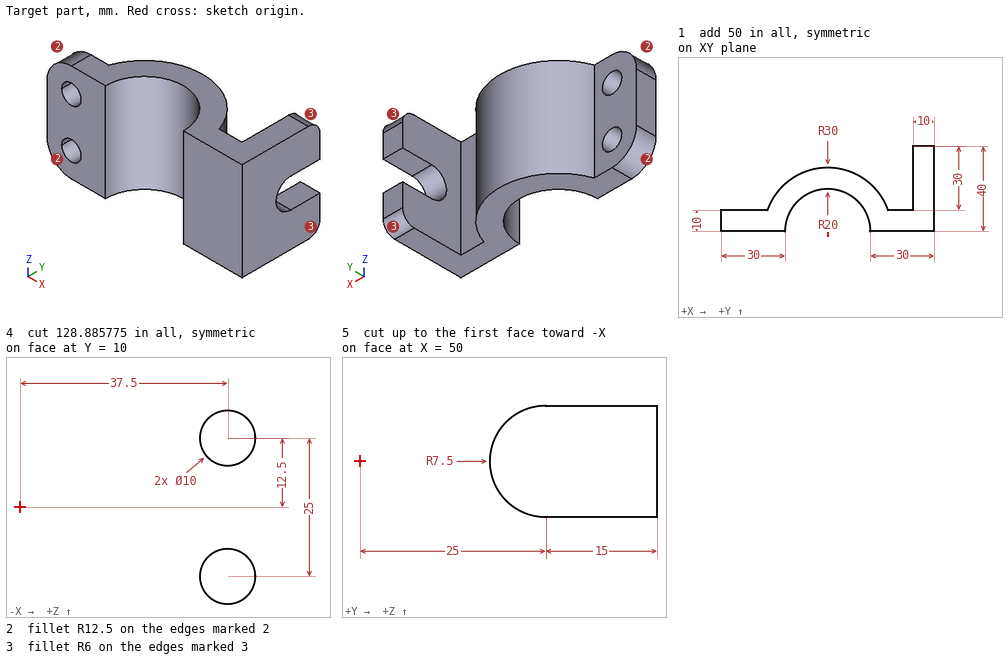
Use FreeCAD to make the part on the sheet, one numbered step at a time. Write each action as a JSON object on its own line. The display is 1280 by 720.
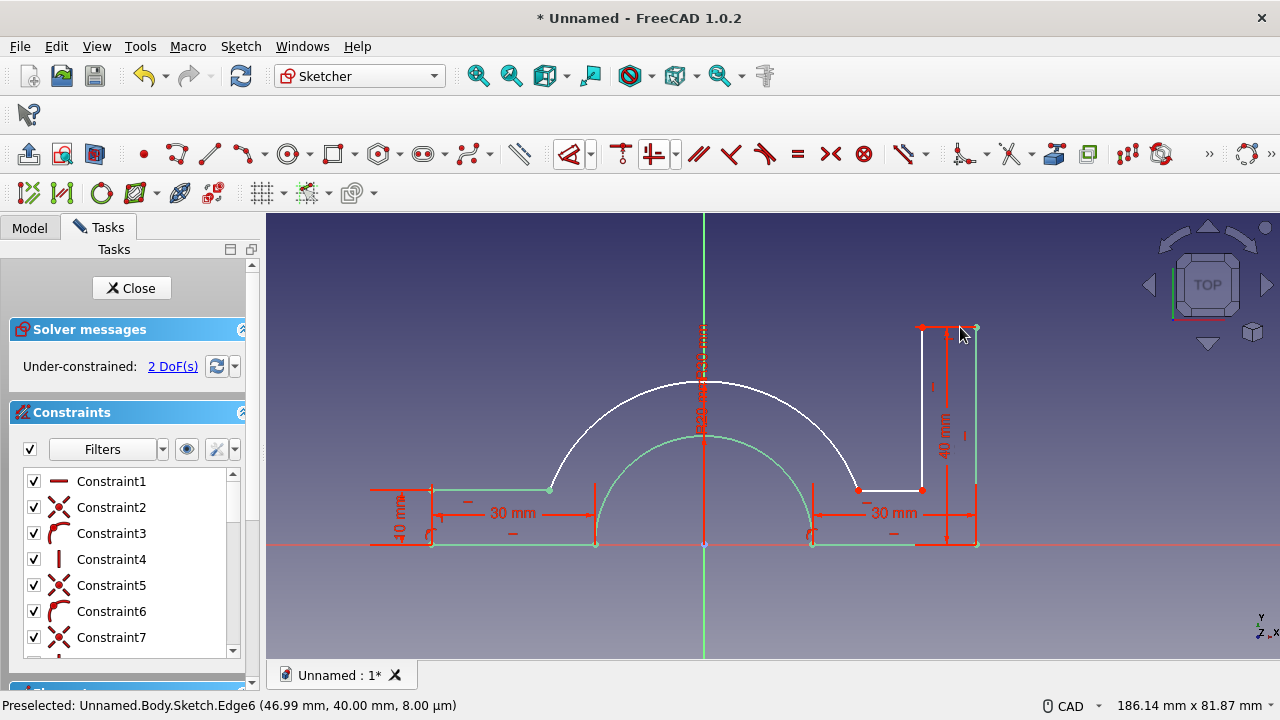
{"action": "key", "text": "l"}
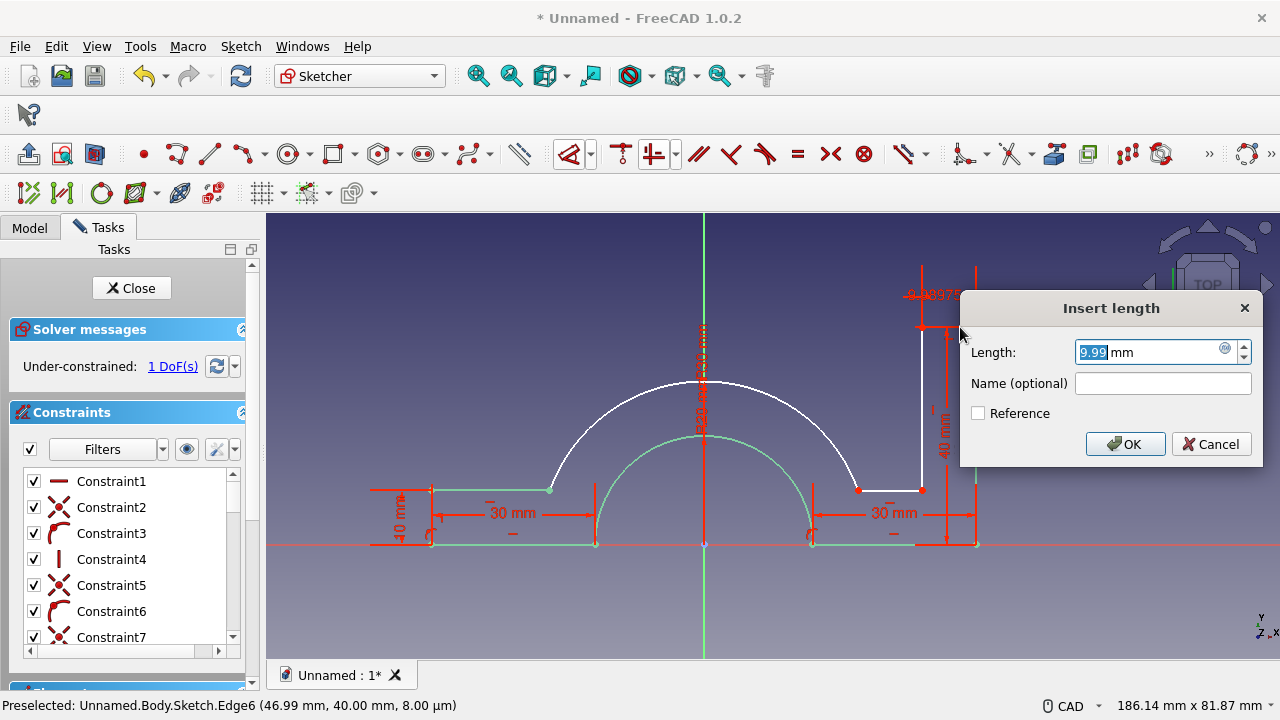
{"action": "type", "text": "10"}
{"action": "key", "text": "Return"}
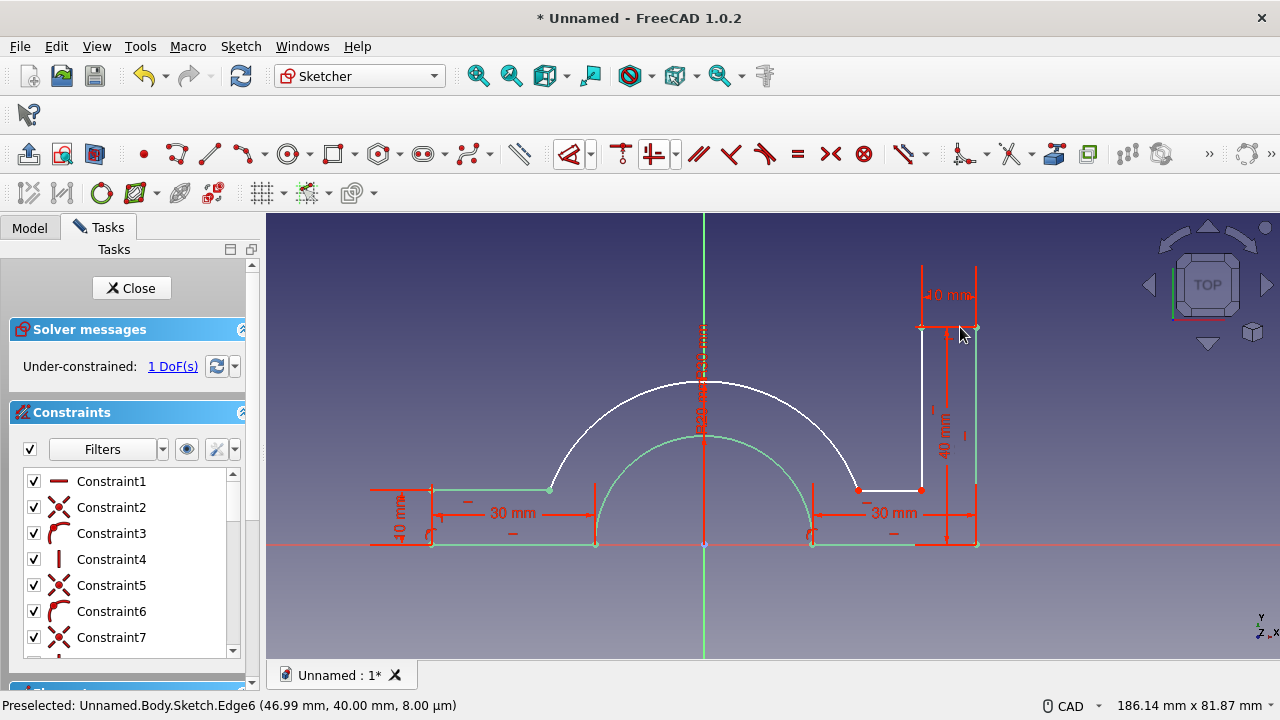
{"action": "left_click", "coordinate": [922, 376]}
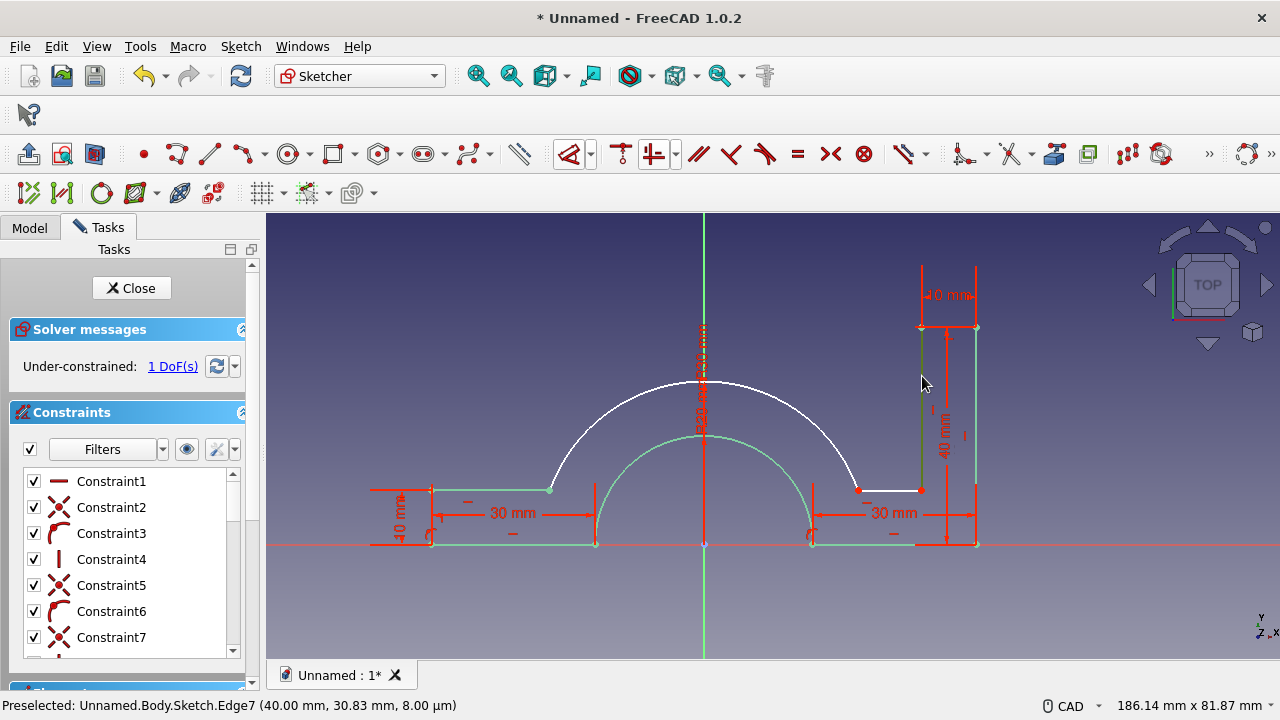
{"action": "left_click", "coordinate": [590, 154]}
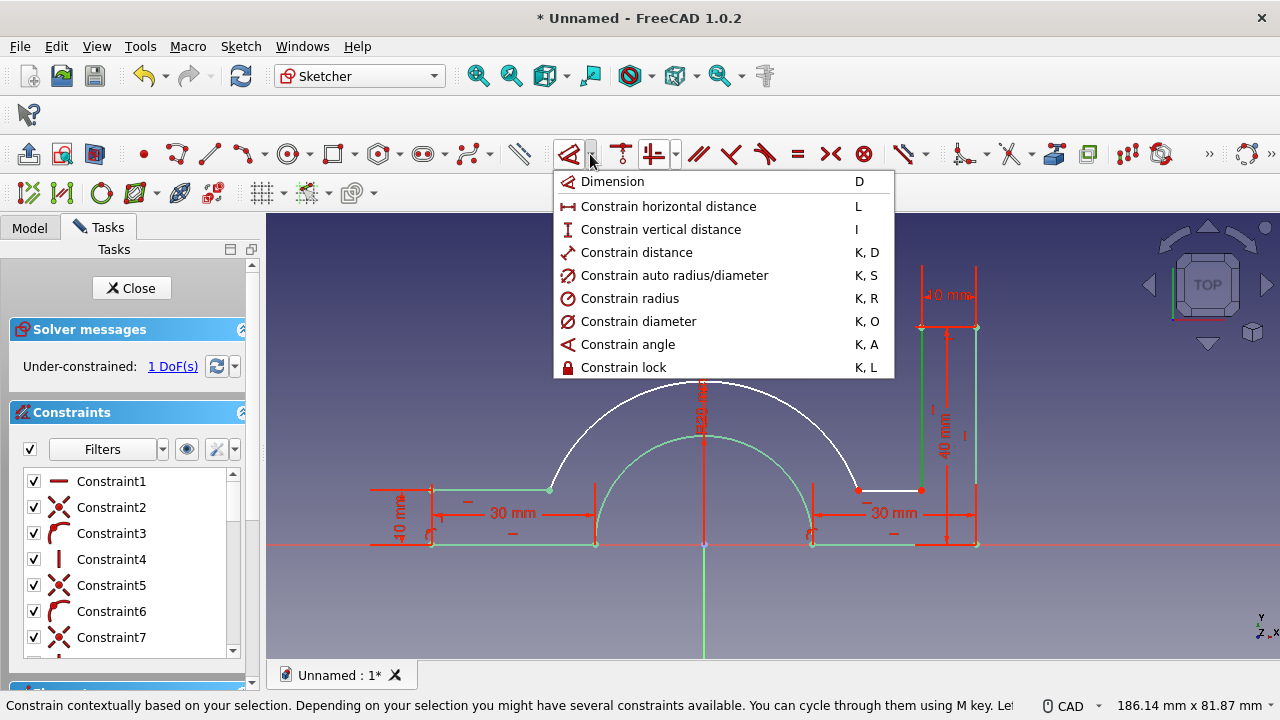
{"action": "left_click", "coordinate": [724, 230]}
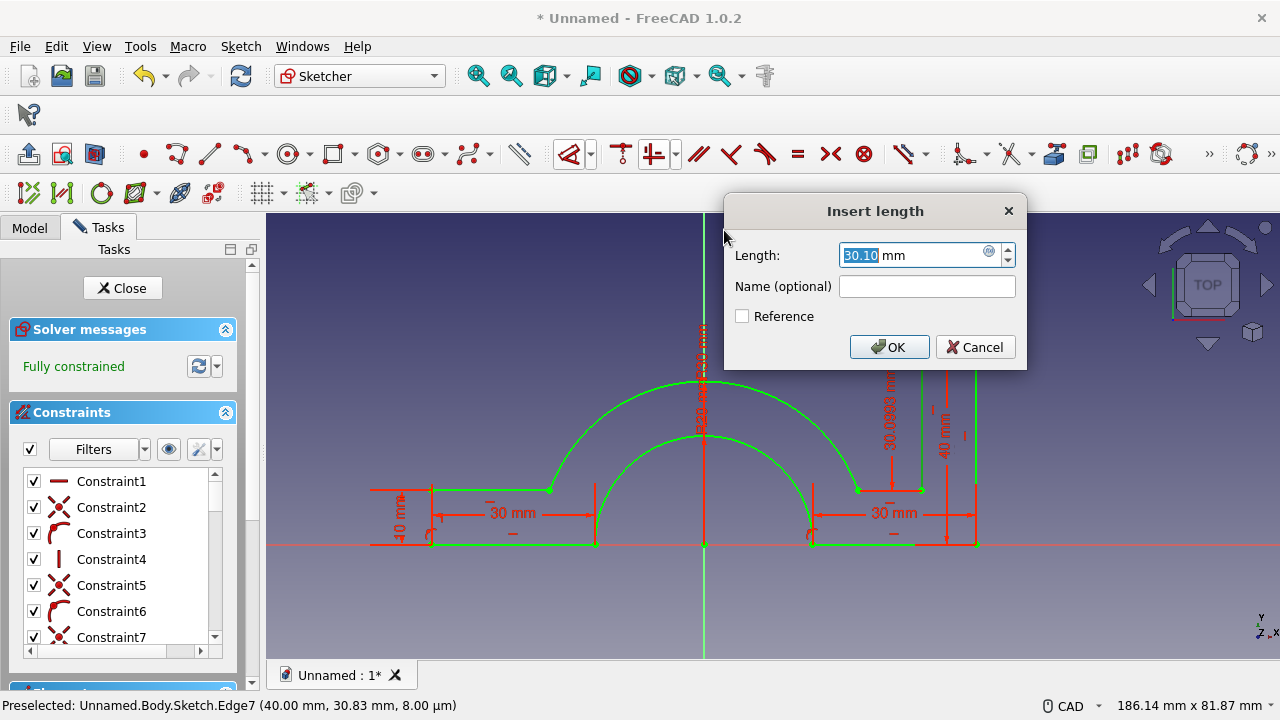
{"action": "type", "text": "30"}
{"action": "key", "text": "Return"}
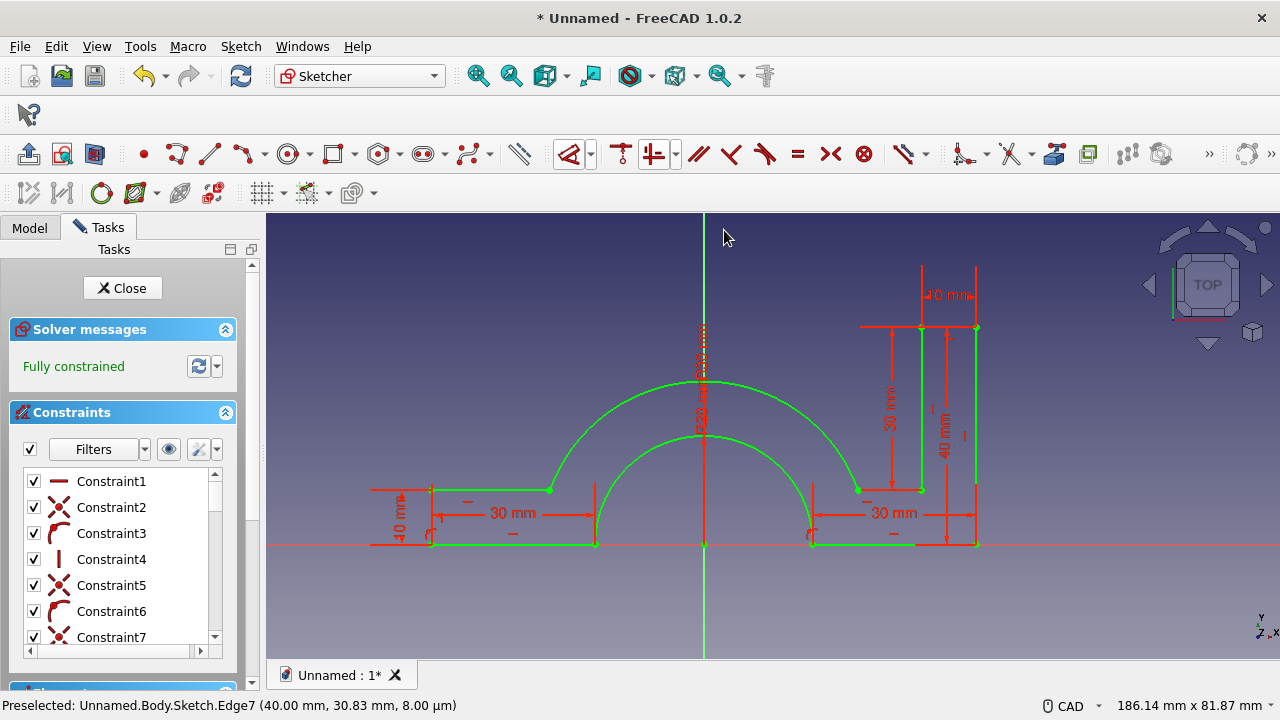
{"action": "left_click", "coordinate": [123, 288]}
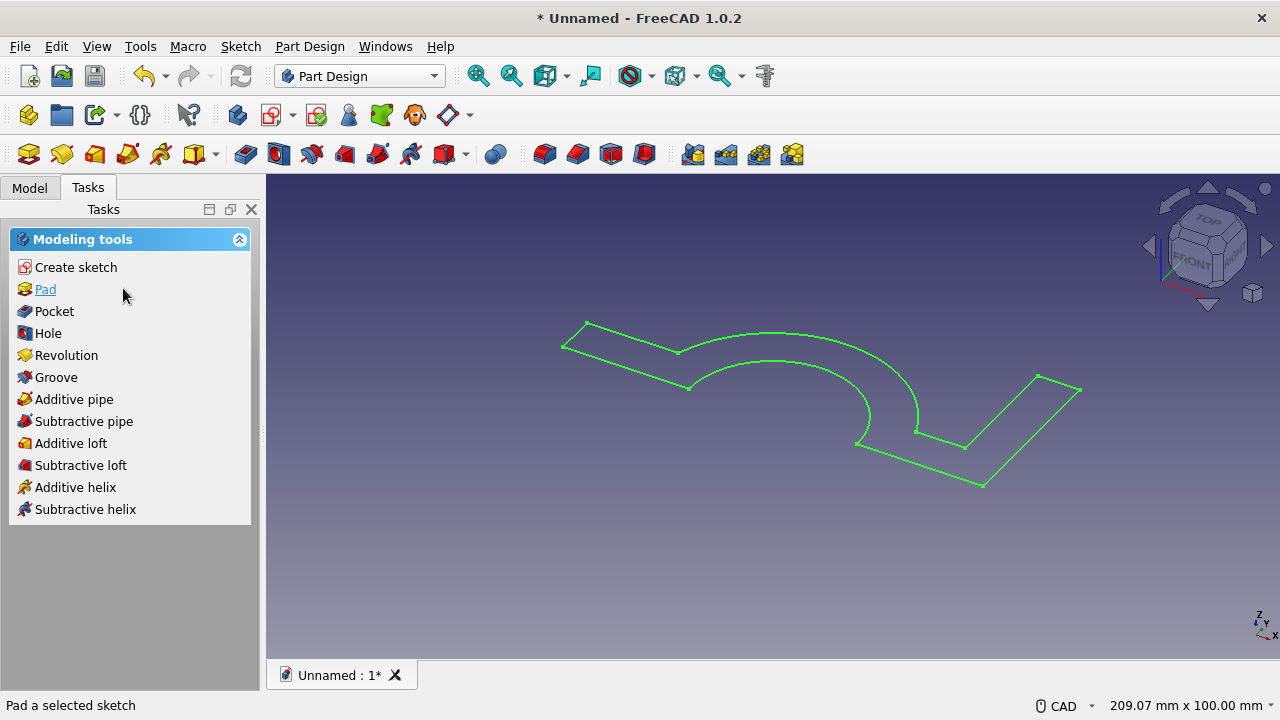
{"action": "left_click", "coordinate": [29, 154]}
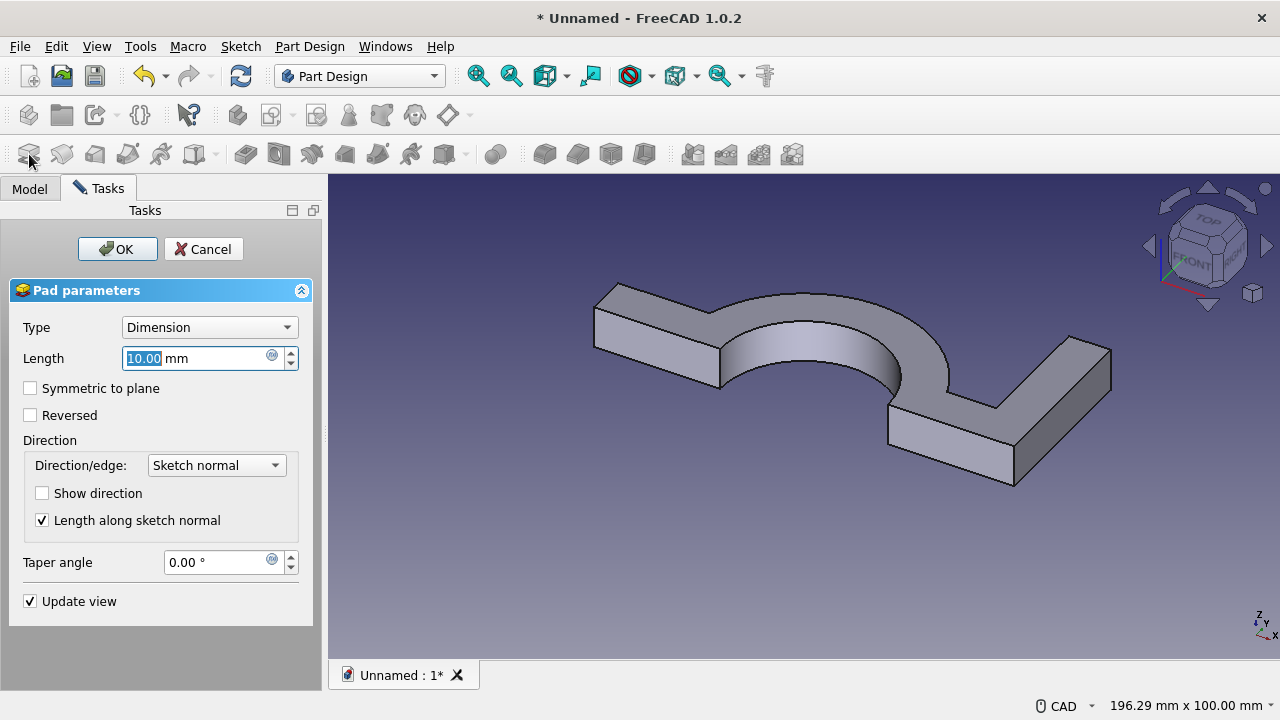
{"action": "type", "text": "50"}
{"action": "key", "text": "Tab"}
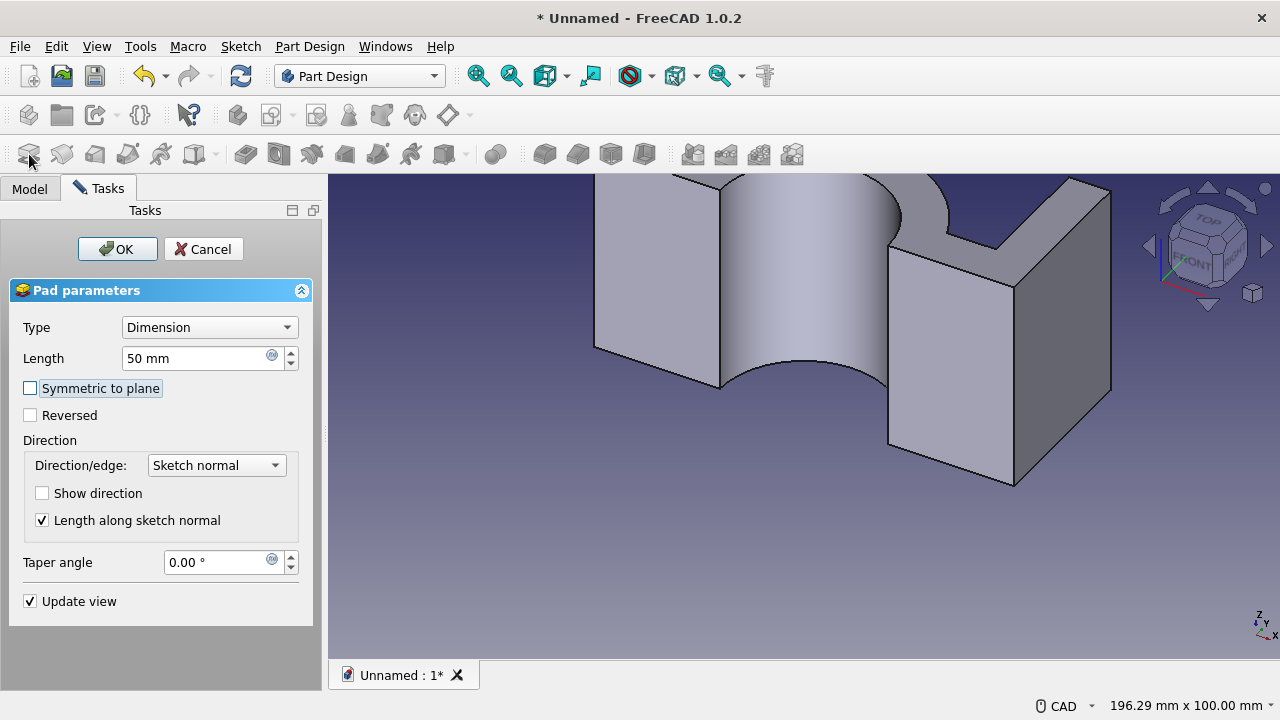
{"action": "left_click", "coordinate": [31, 388]}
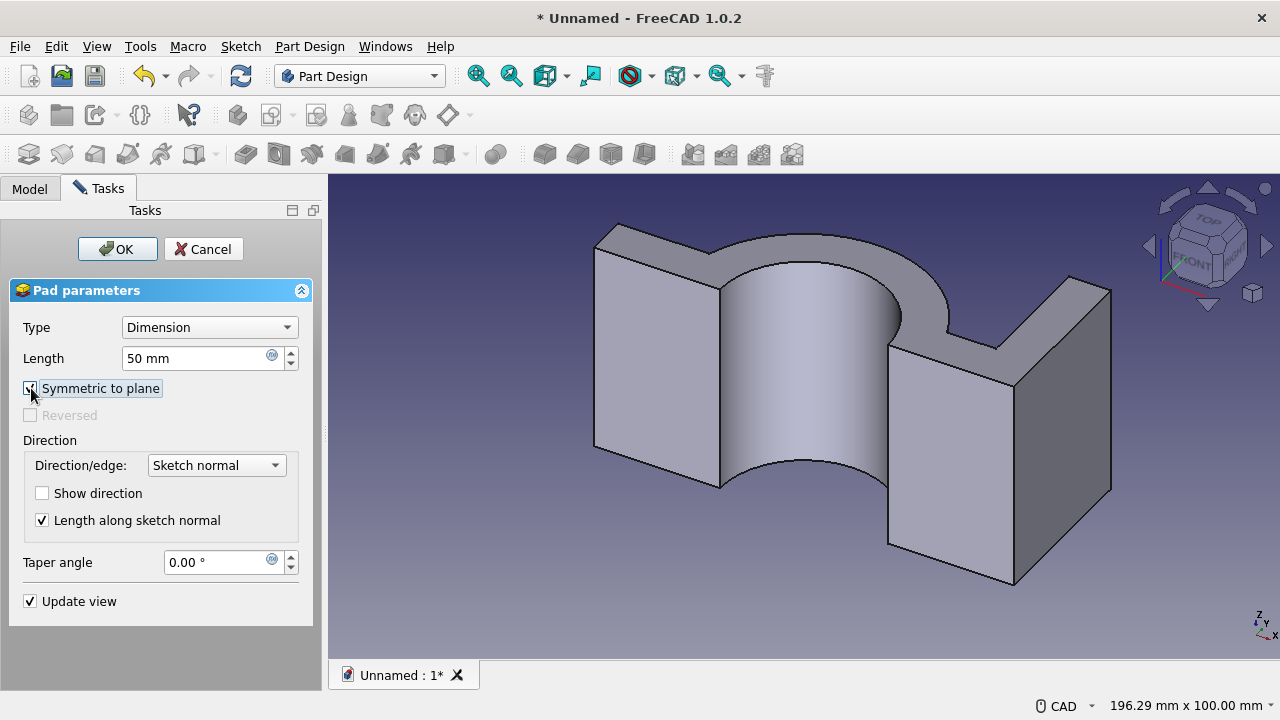
{"action": "left_click", "coordinate": [118, 249]}